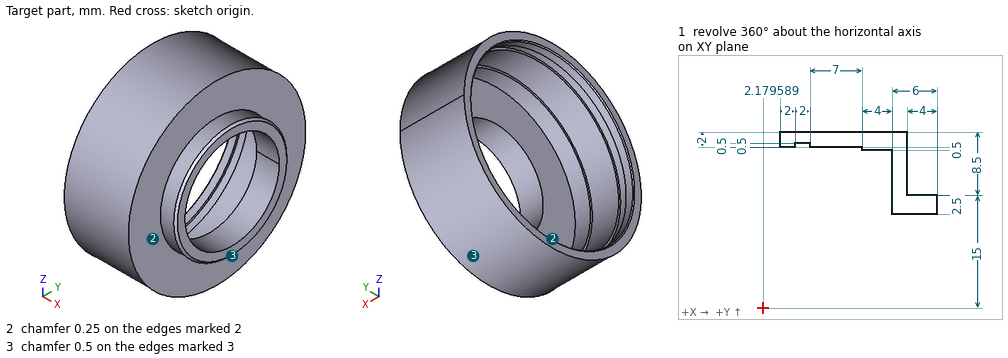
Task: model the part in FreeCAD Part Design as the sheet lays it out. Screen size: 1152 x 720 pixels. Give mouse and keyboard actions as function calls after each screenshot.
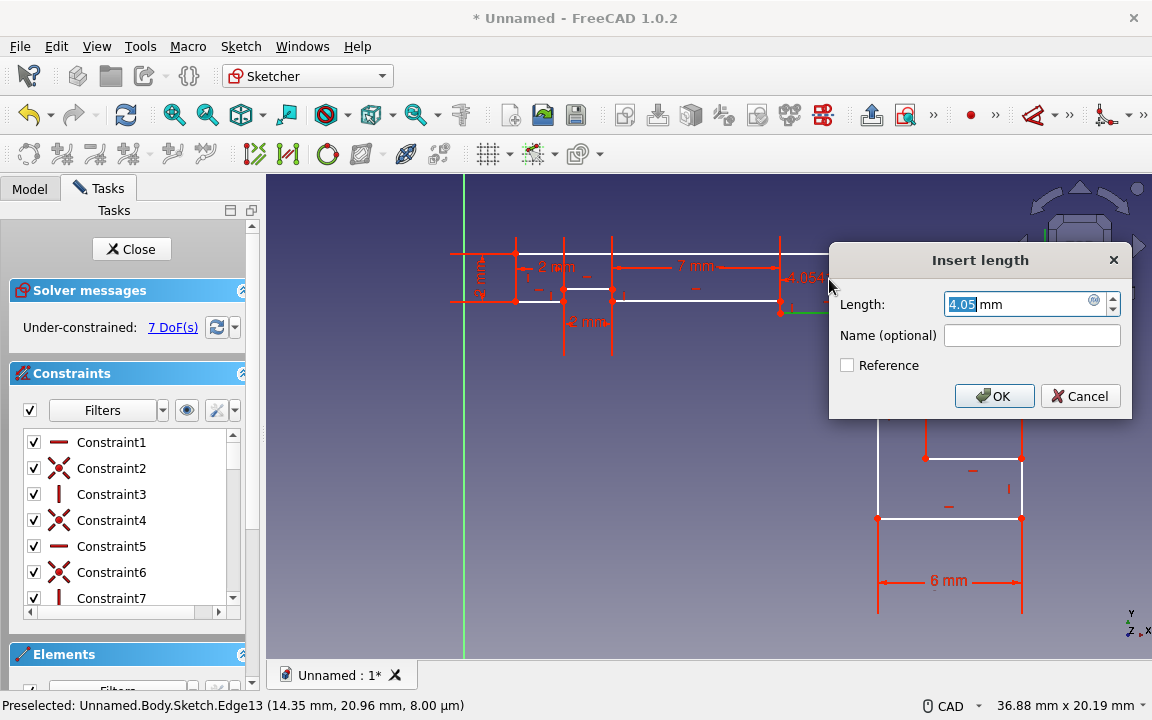
text(4)
key(Return)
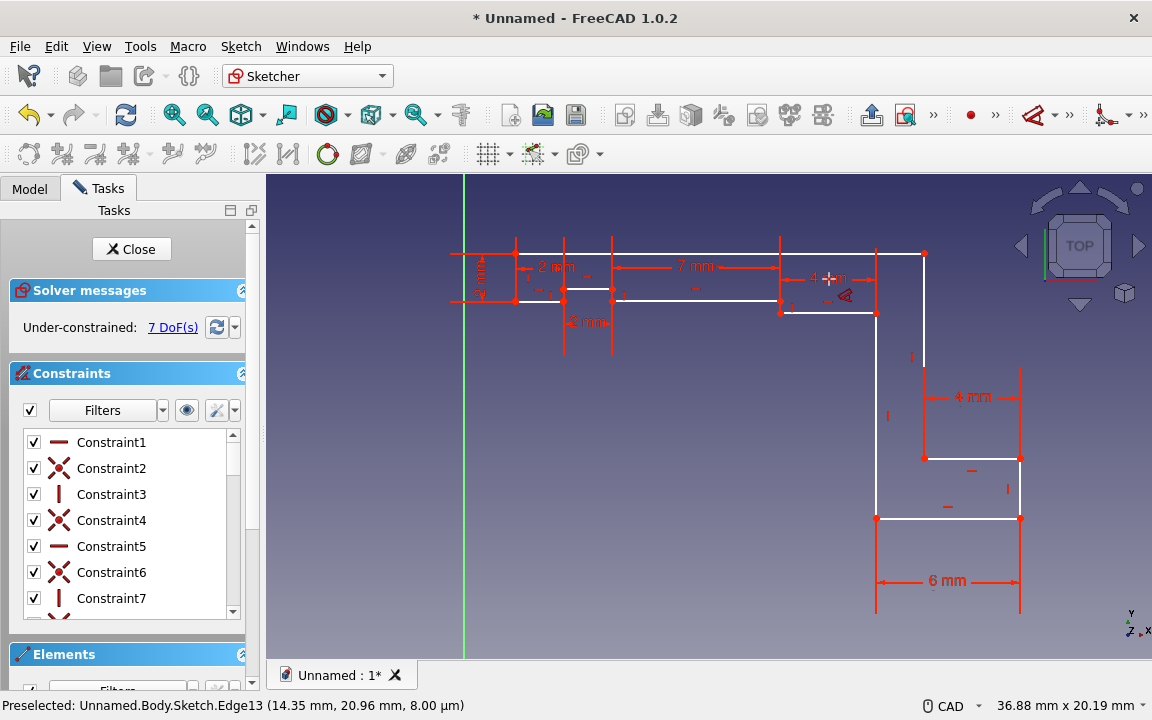
scroll(516, 273, down, 3)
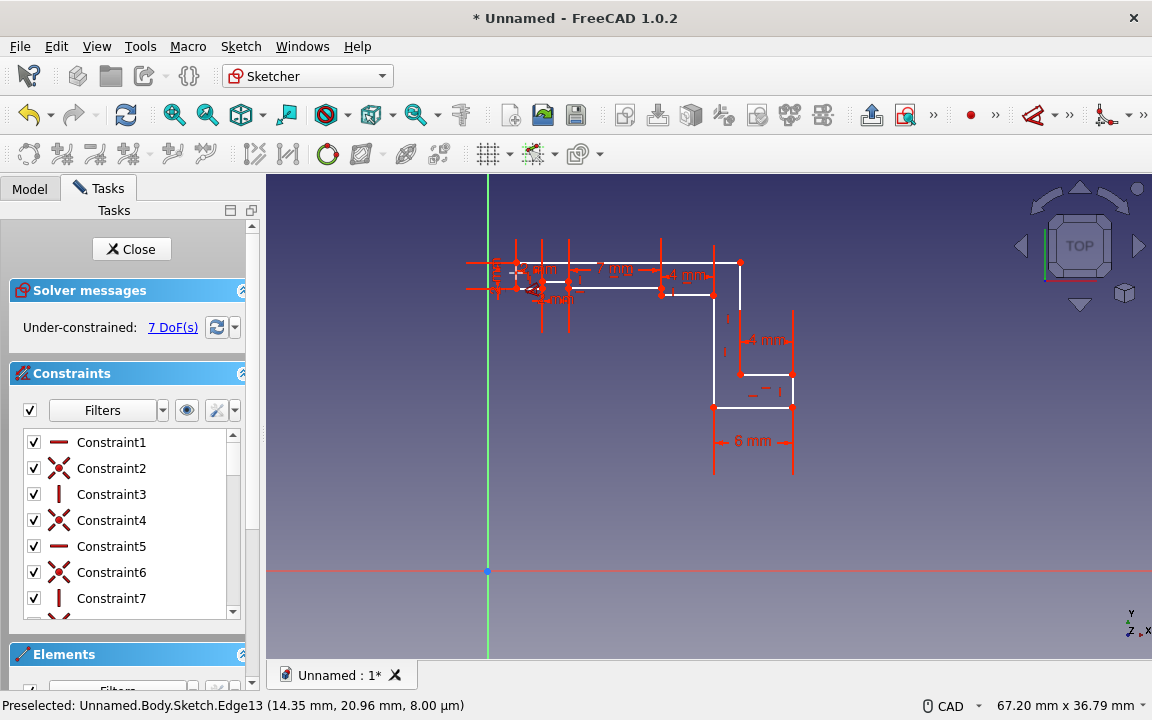
scroll(793, 398, up, 2)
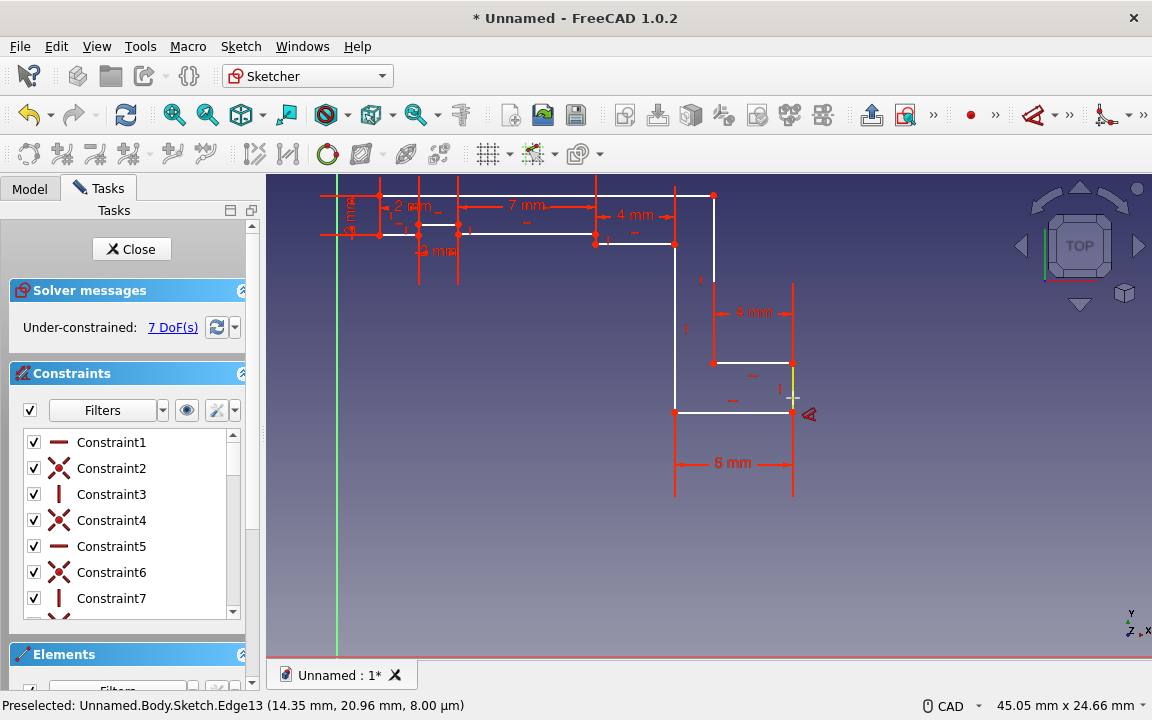
click(793, 398)
click(827, 388)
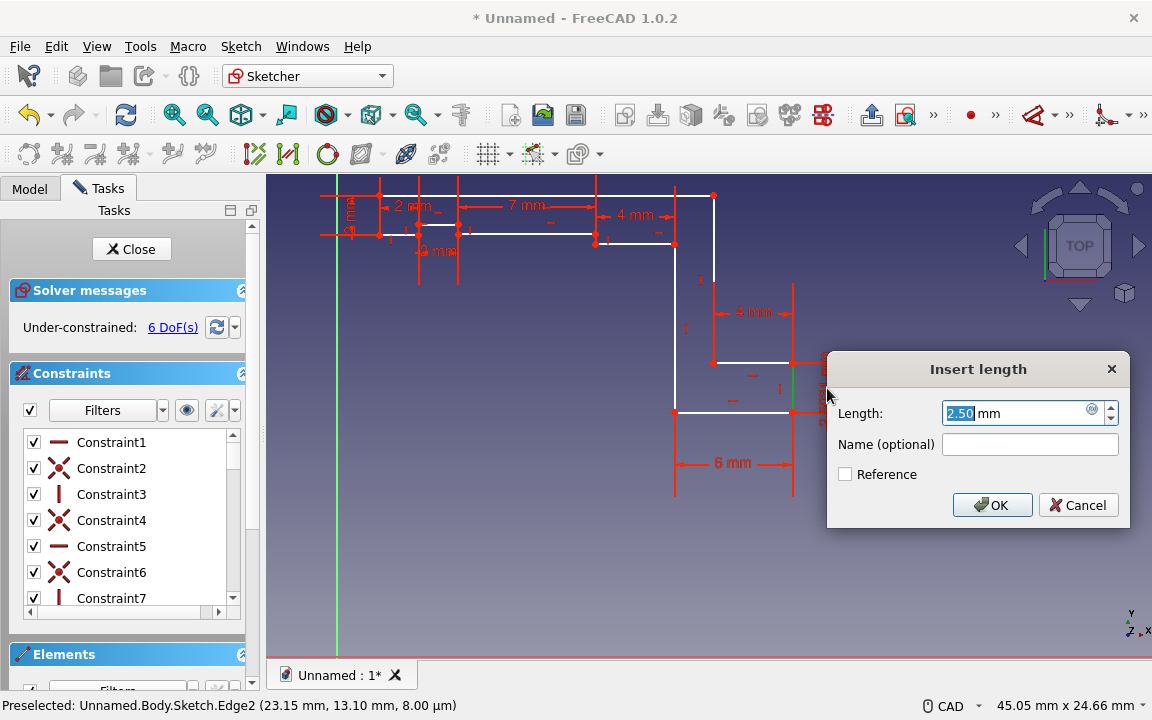
text(2.5)
key(Return)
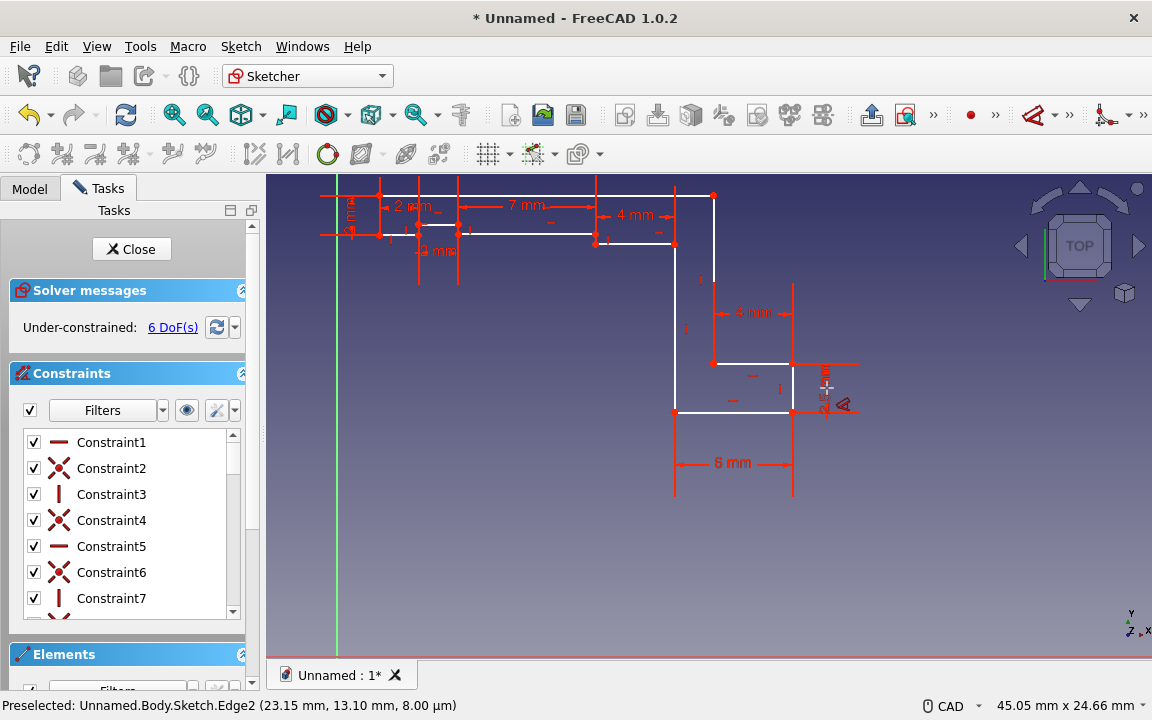
click(714, 313)
click(748, 283)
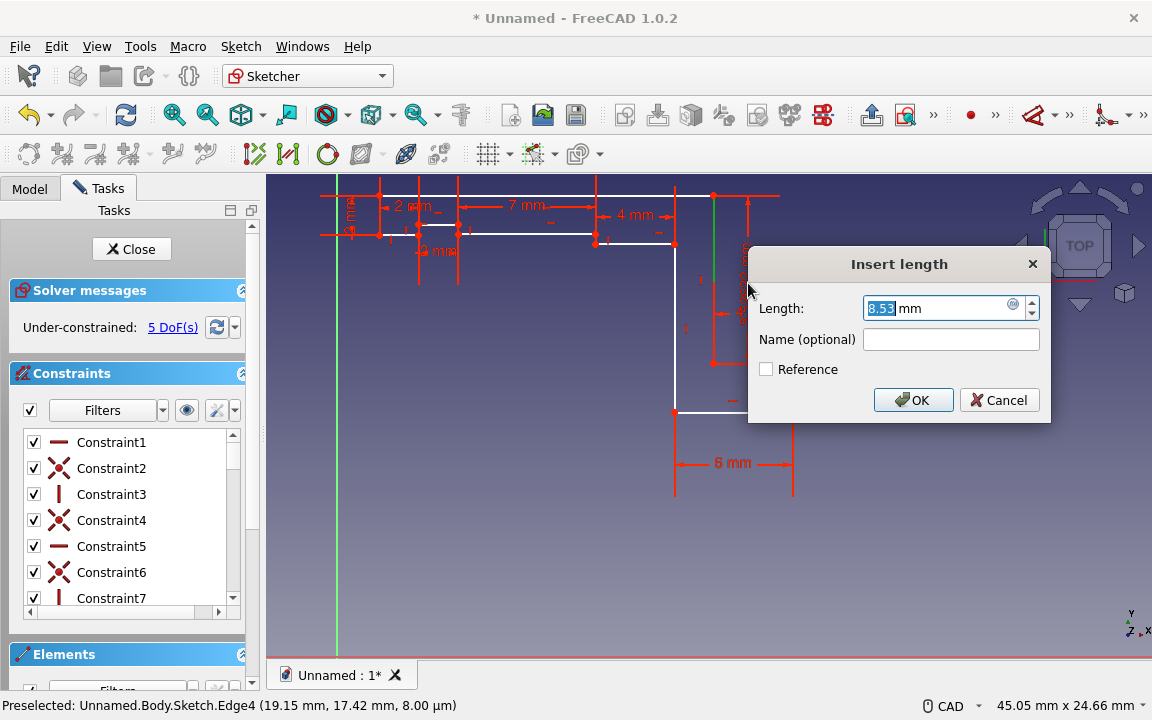
text(8.5)
key(Return)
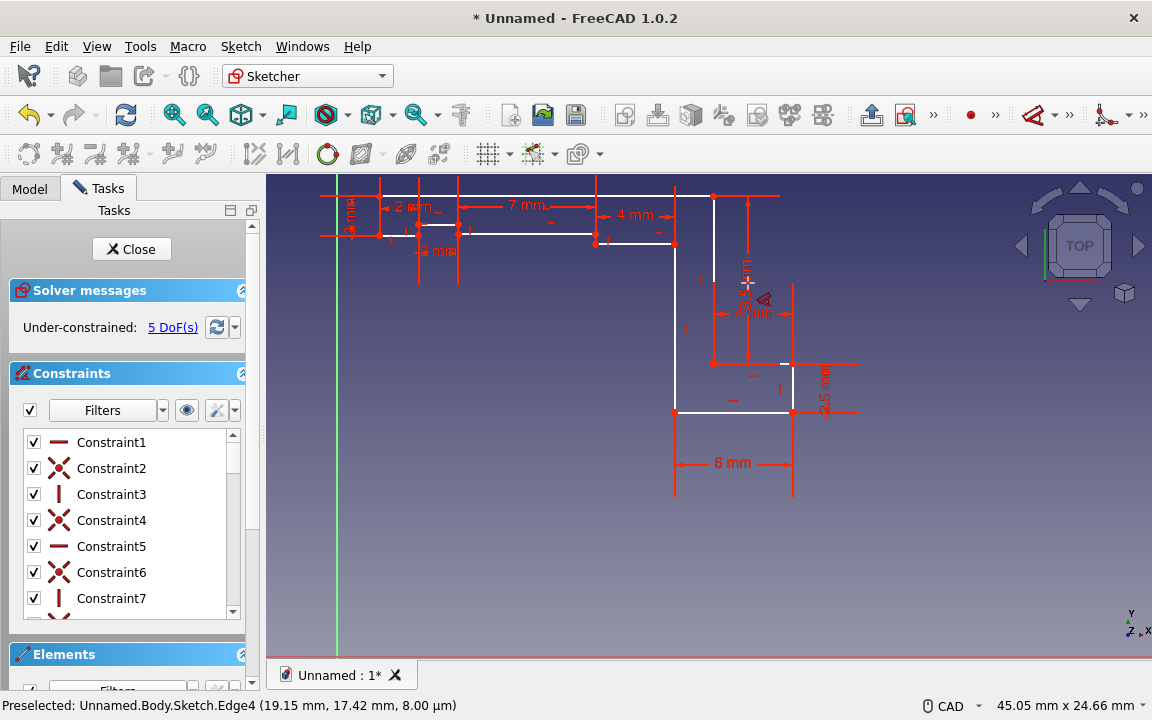
scroll(419, 230, up, 7)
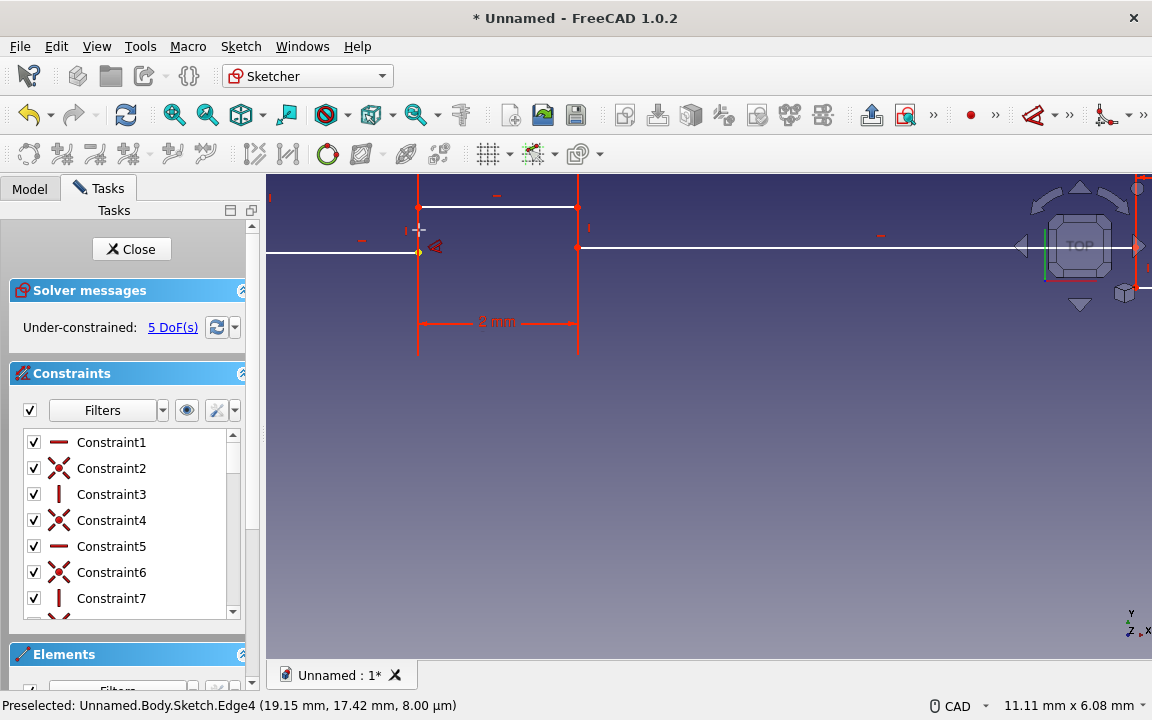
click(418, 230)
click(384, 230)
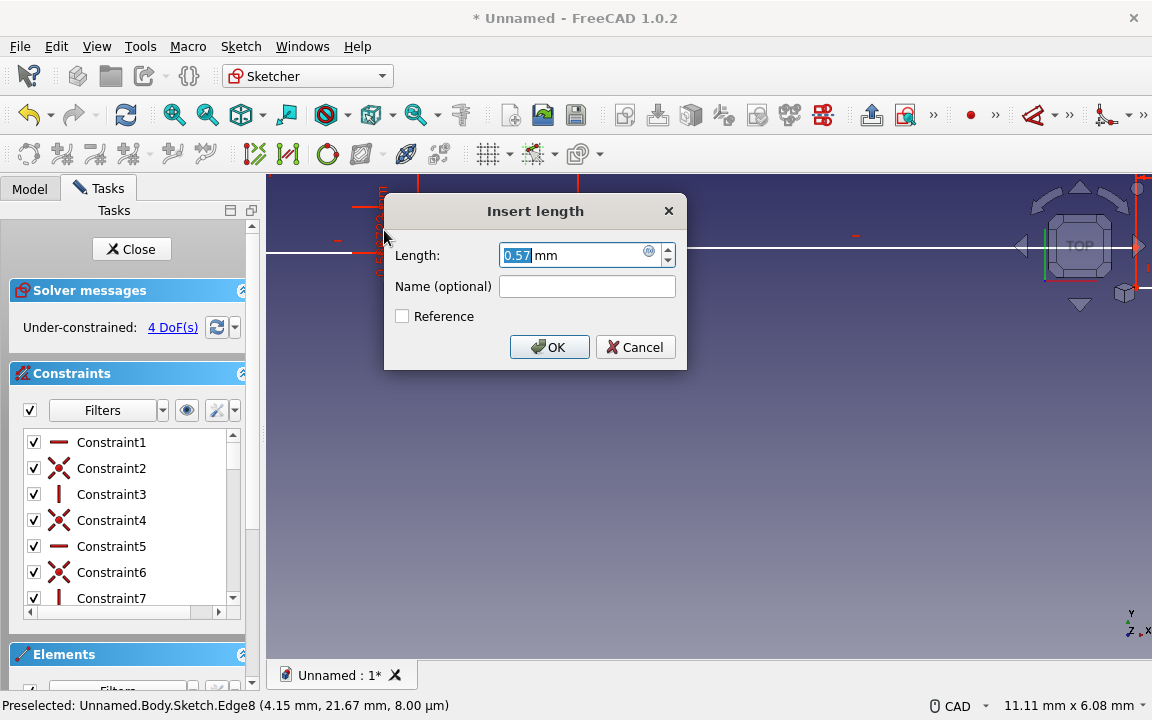
text(0.5)
key(Return)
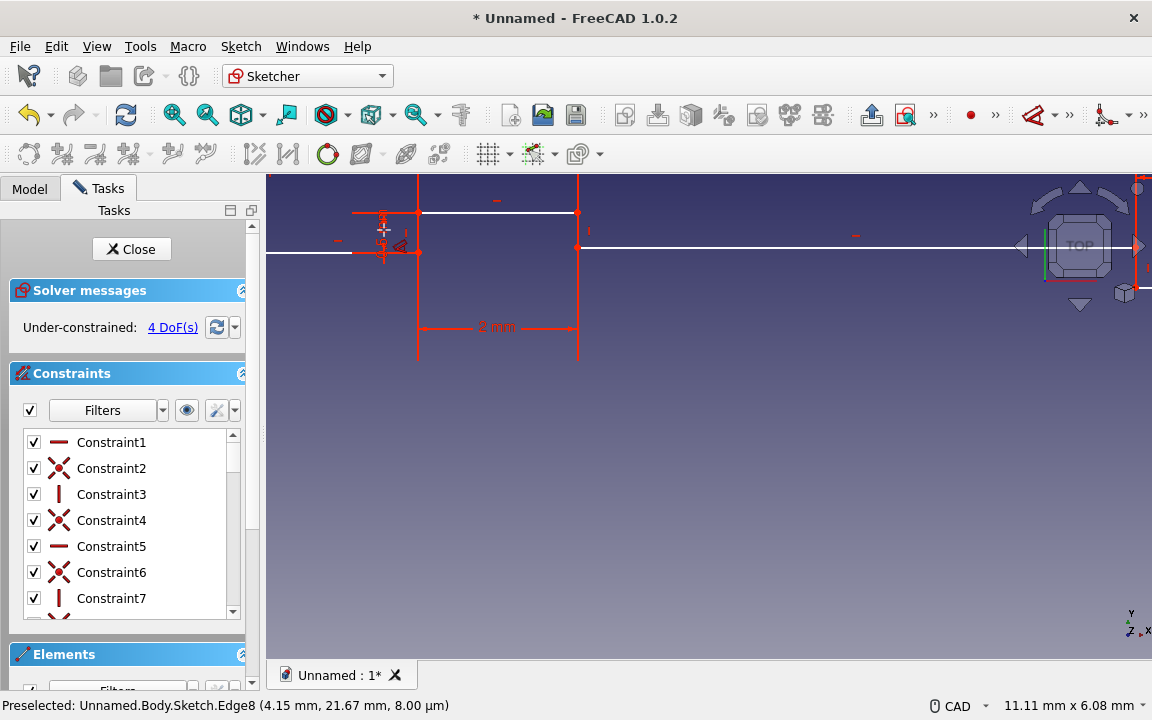
scroll(578, 223, up, 2)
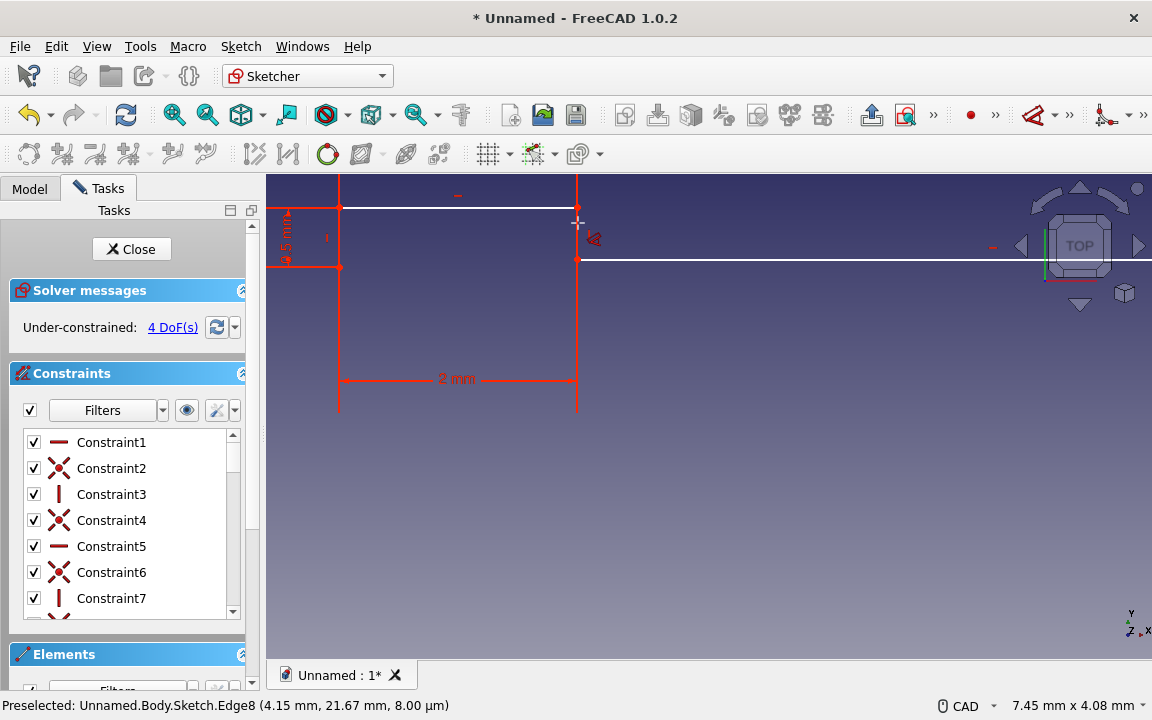
click(577, 223)
click(543, 234)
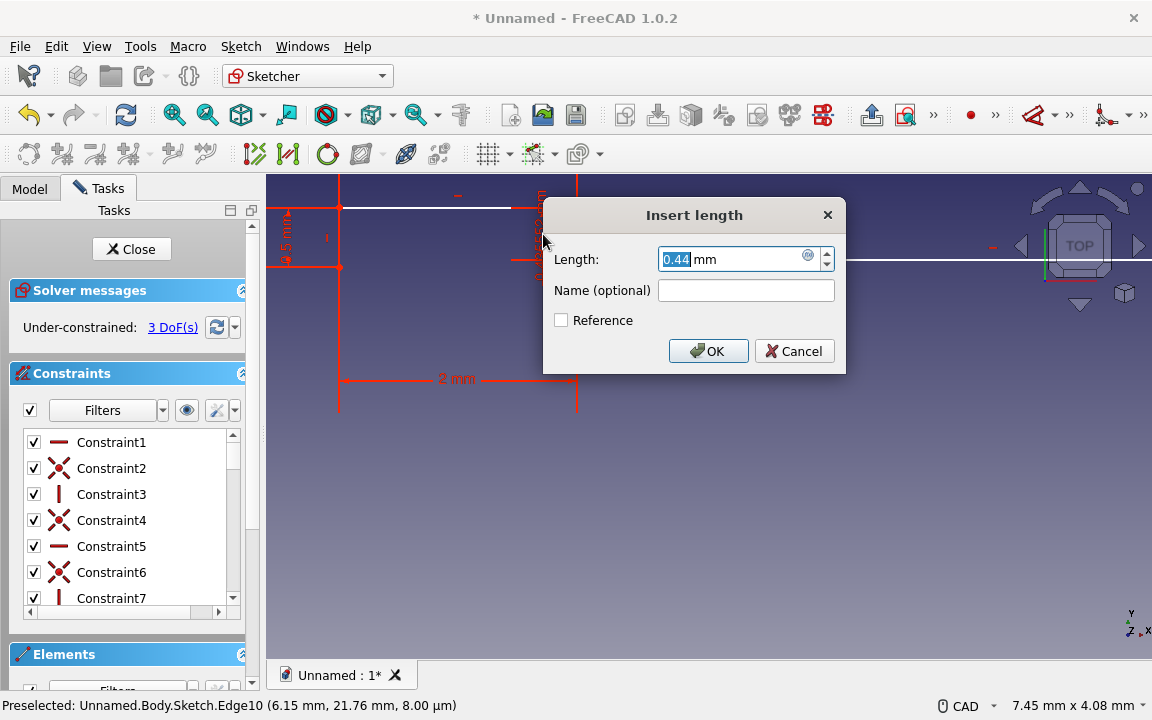
text(0.5)
key(Return)